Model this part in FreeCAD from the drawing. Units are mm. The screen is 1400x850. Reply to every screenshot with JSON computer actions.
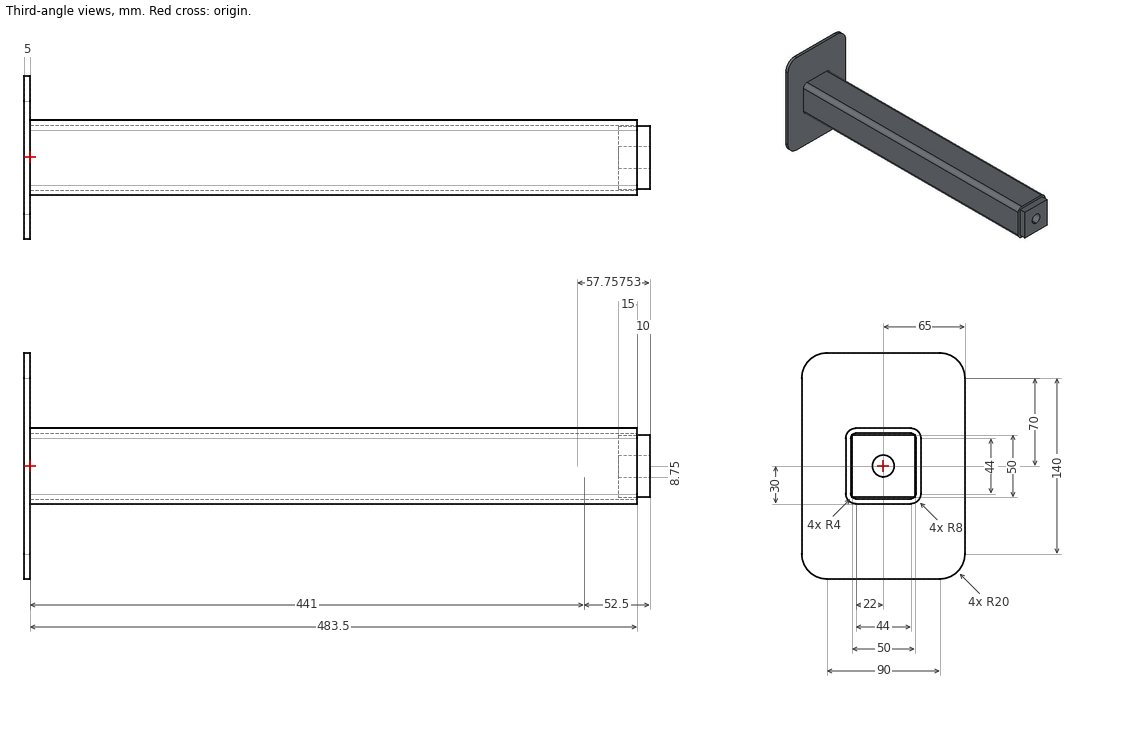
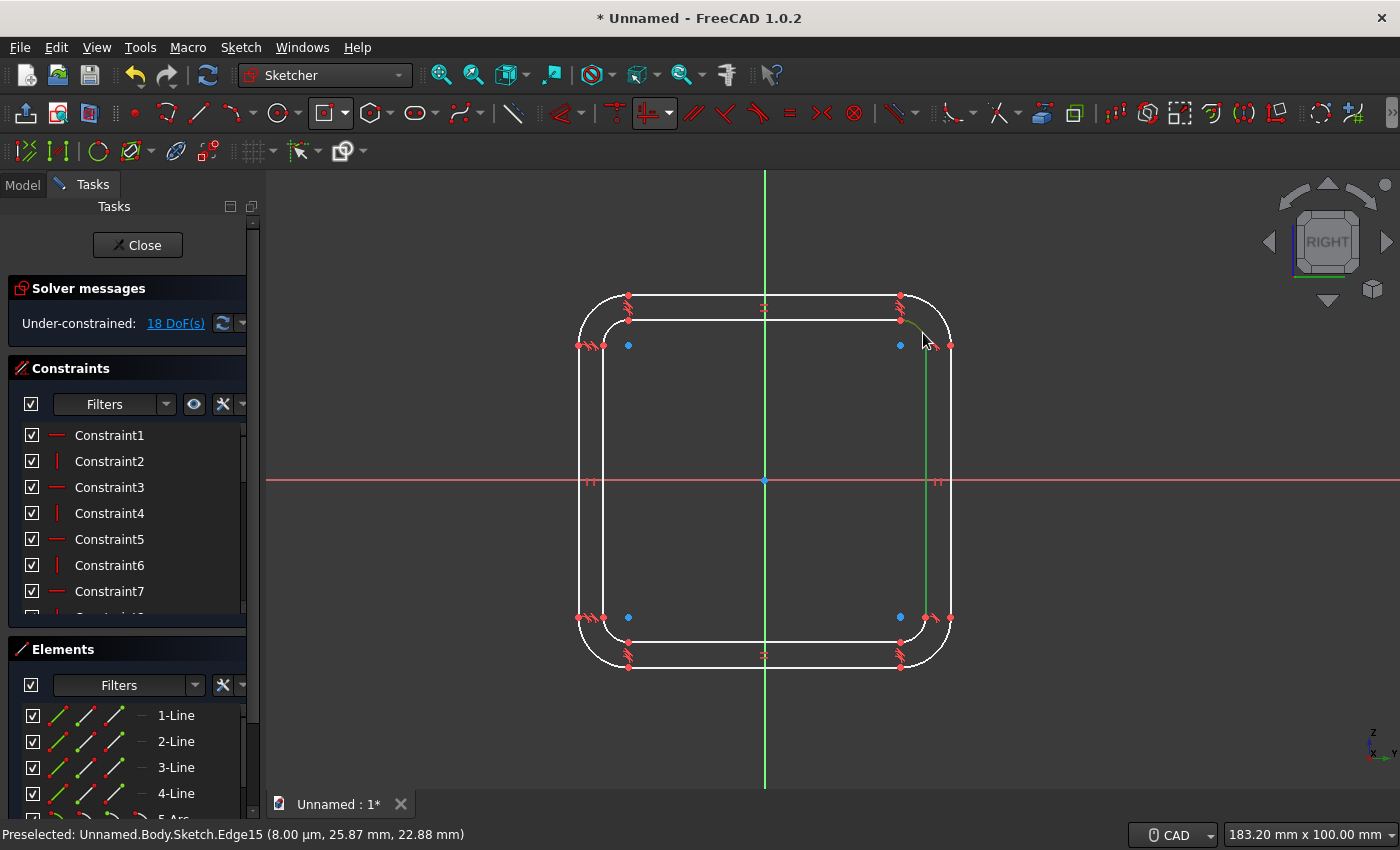
{"action": "key", "text": "t"}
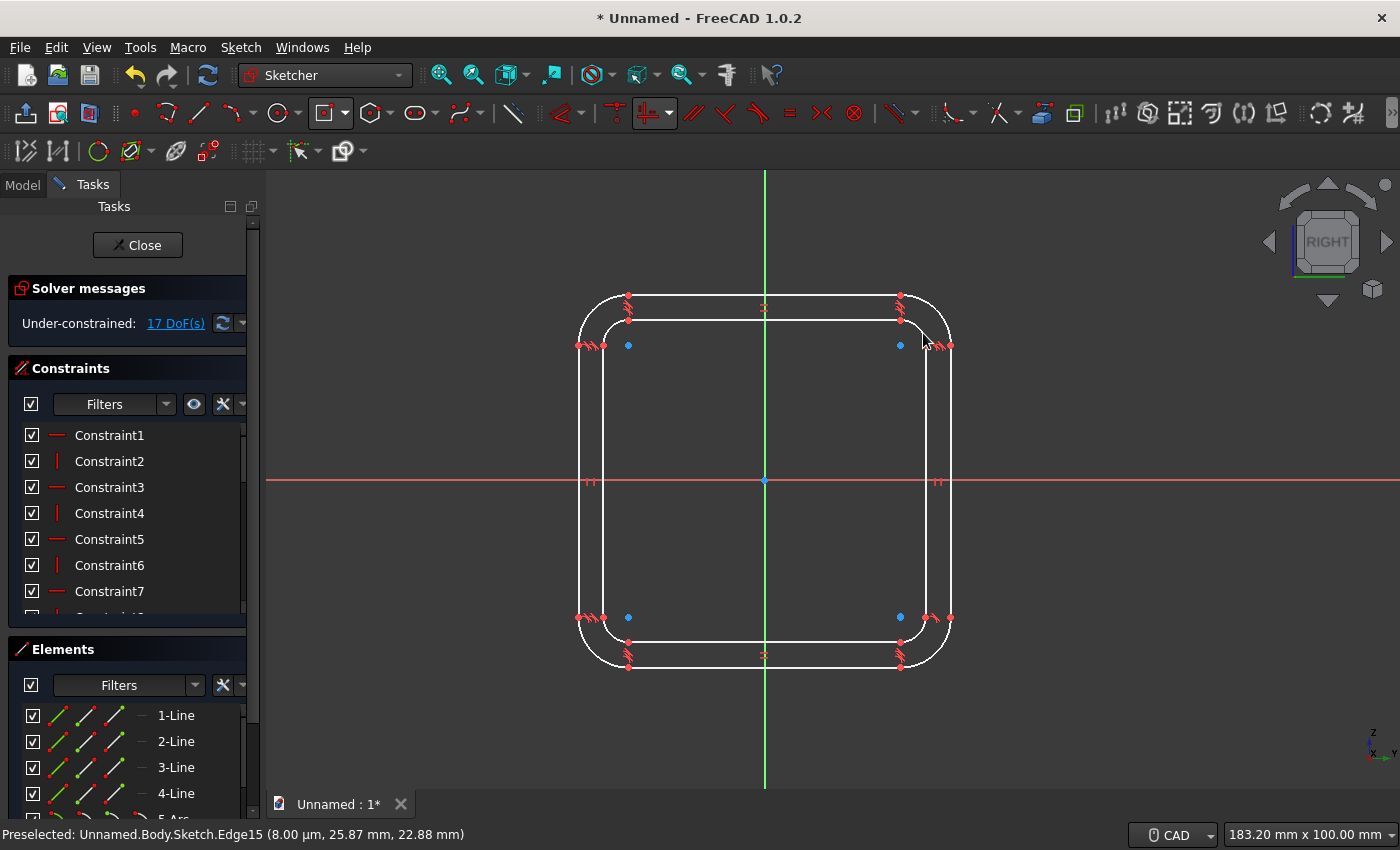
{"action": "left_click", "coordinate": [926, 427]}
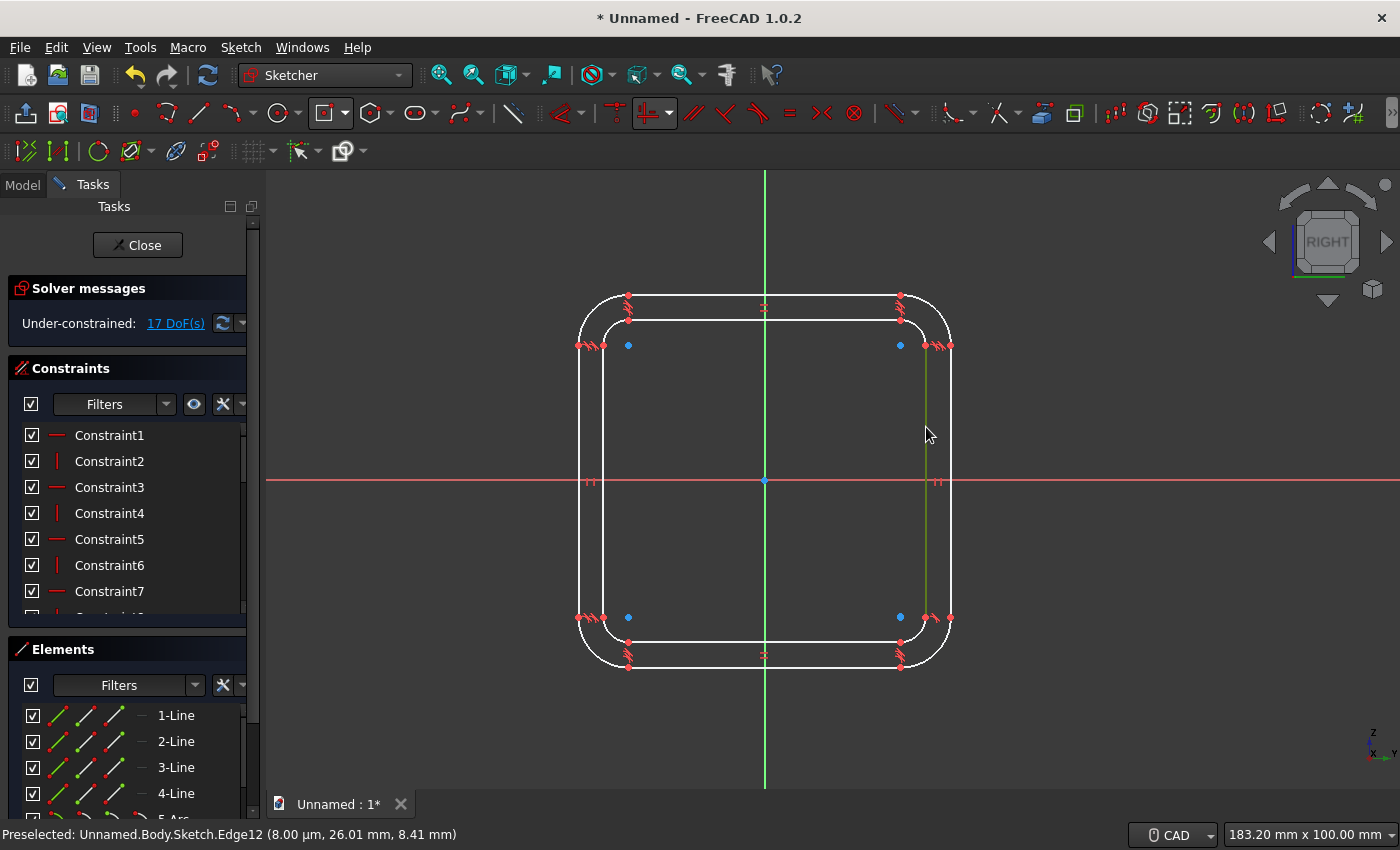
{"action": "left_click", "coordinate": [912, 639]}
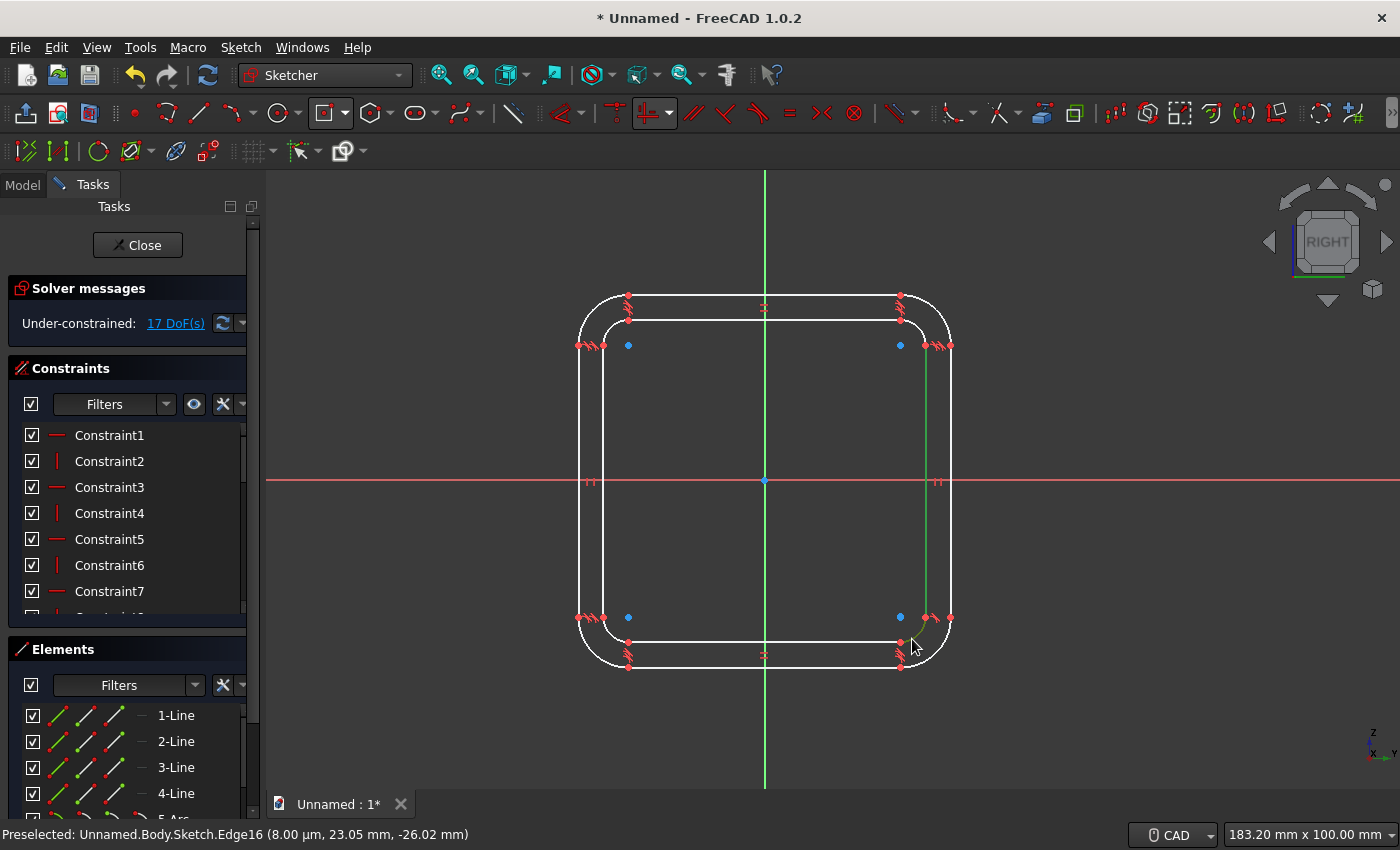
{"action": "left_click", "coordinate": [758, 114]}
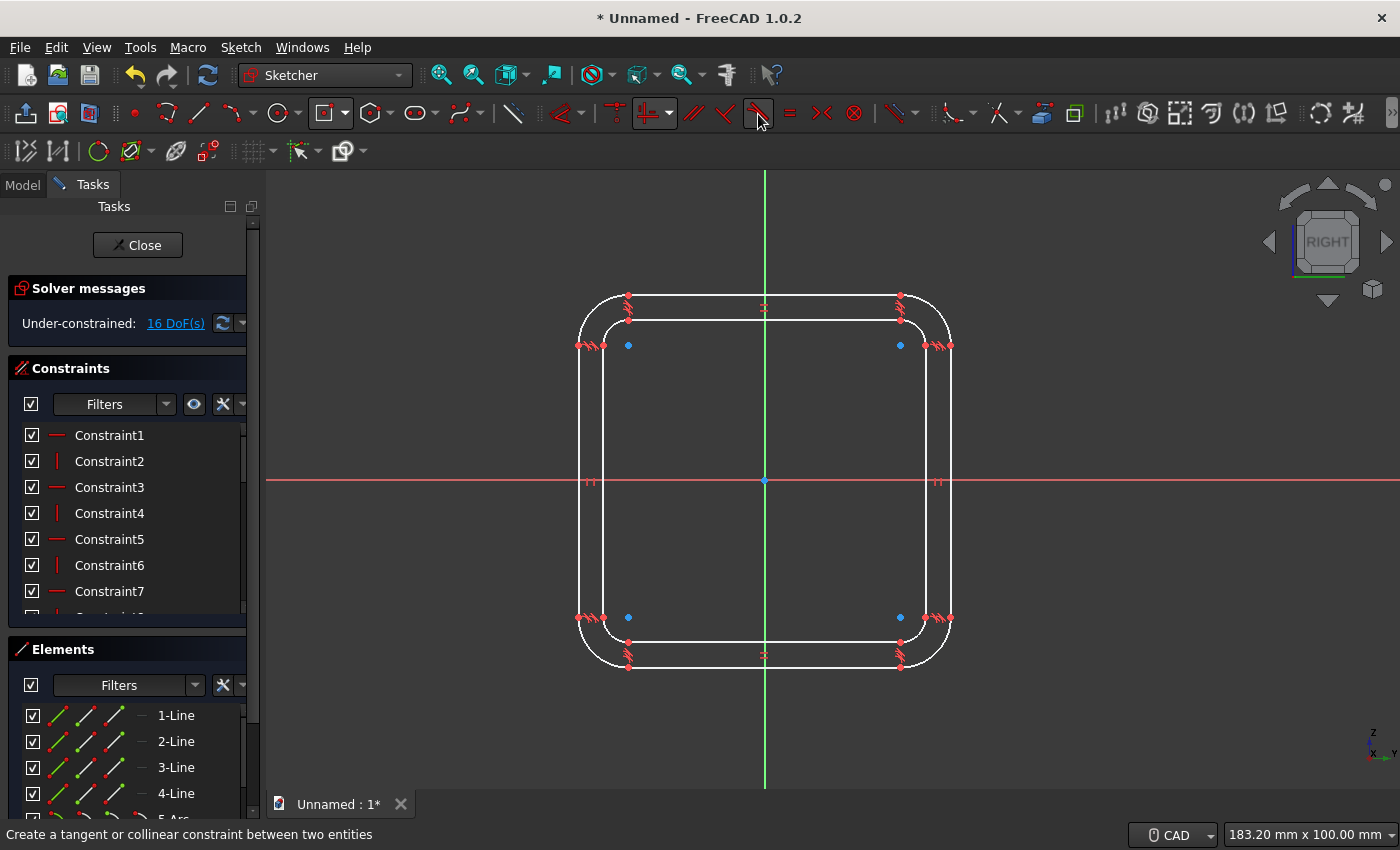
{"action": "left_click", "coordinate": [584, 640]}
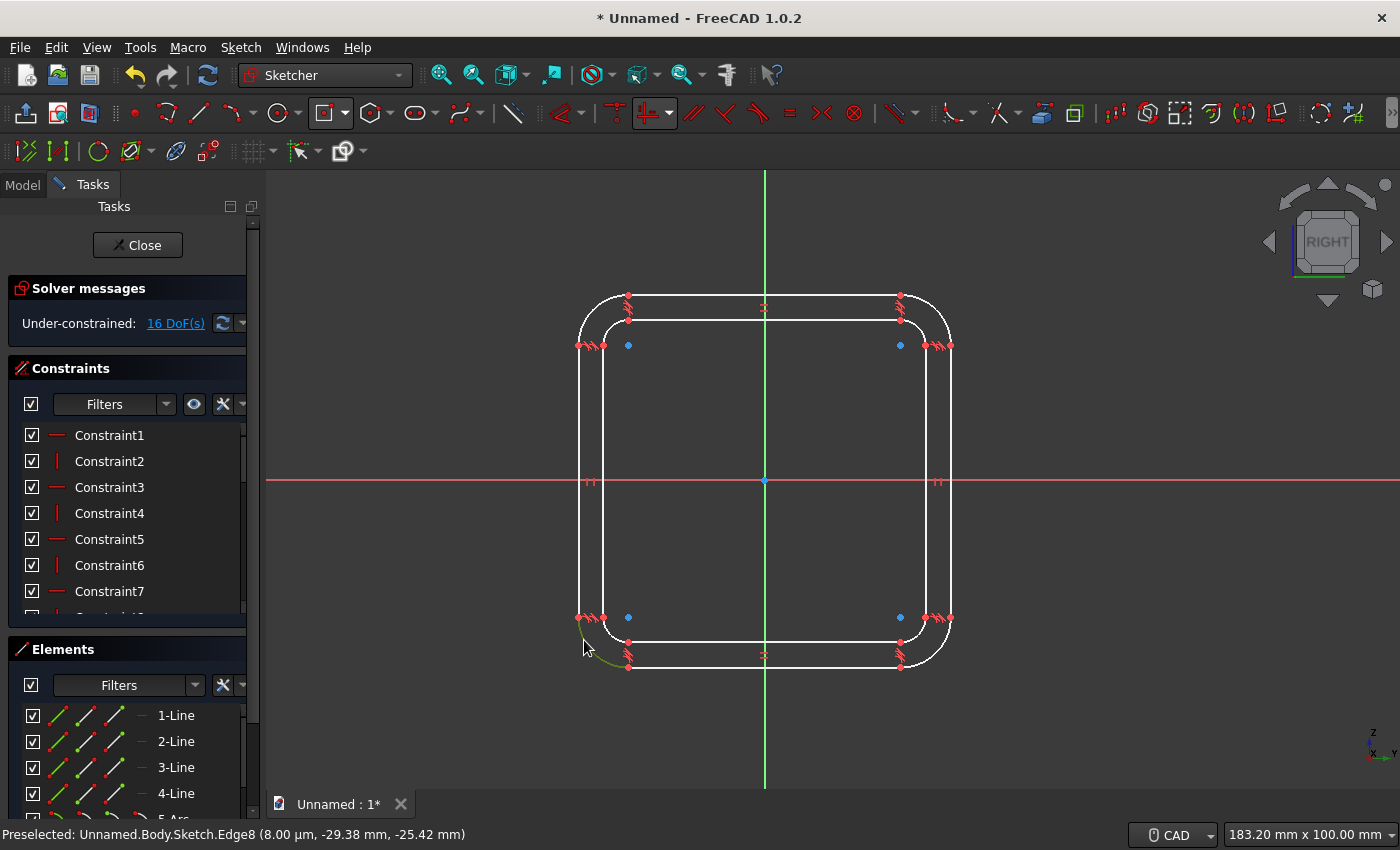
{"action": "left_click", "coordinate": [606, 629]}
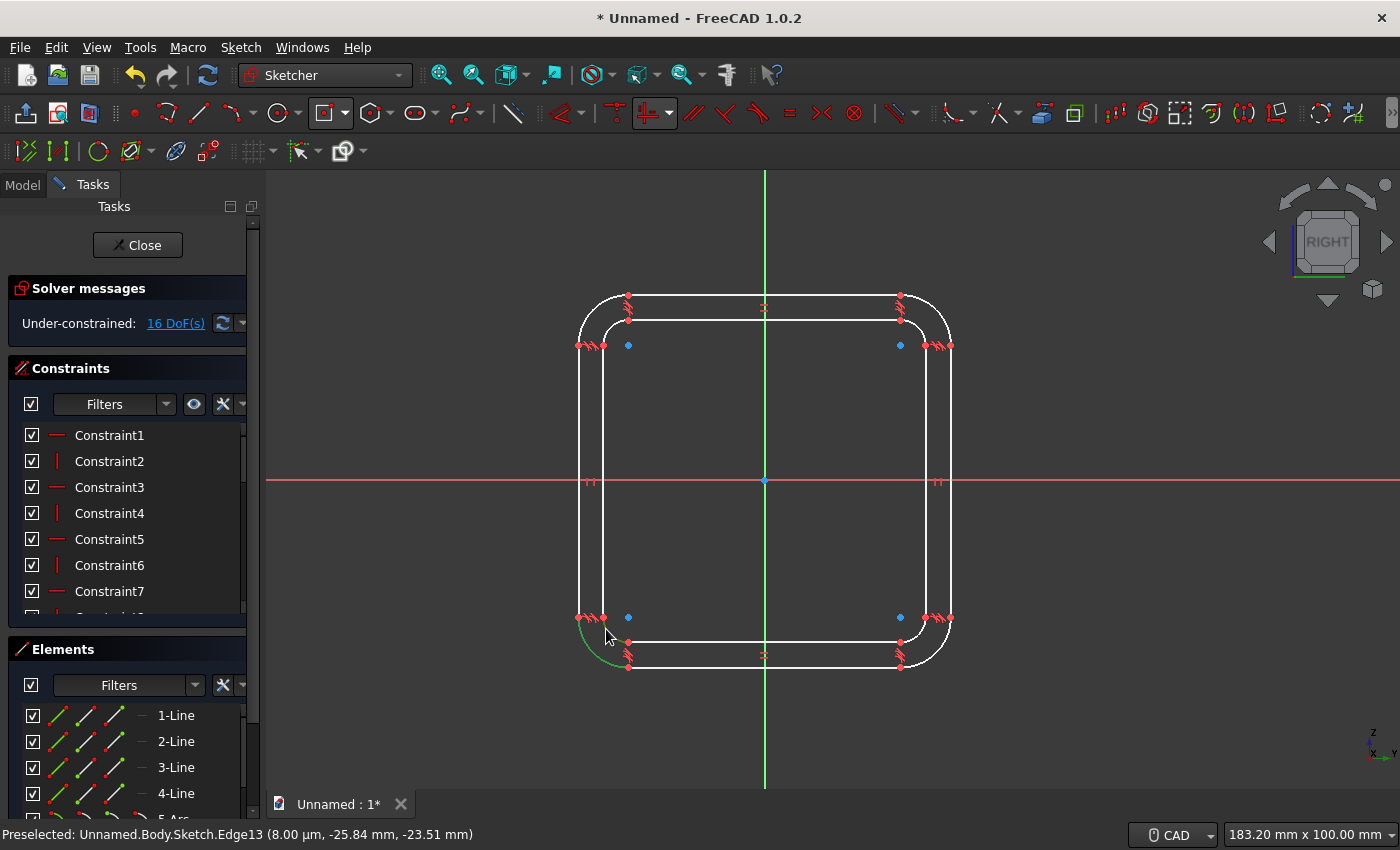
{"action": "left_click", "coordinate": [616, 114]}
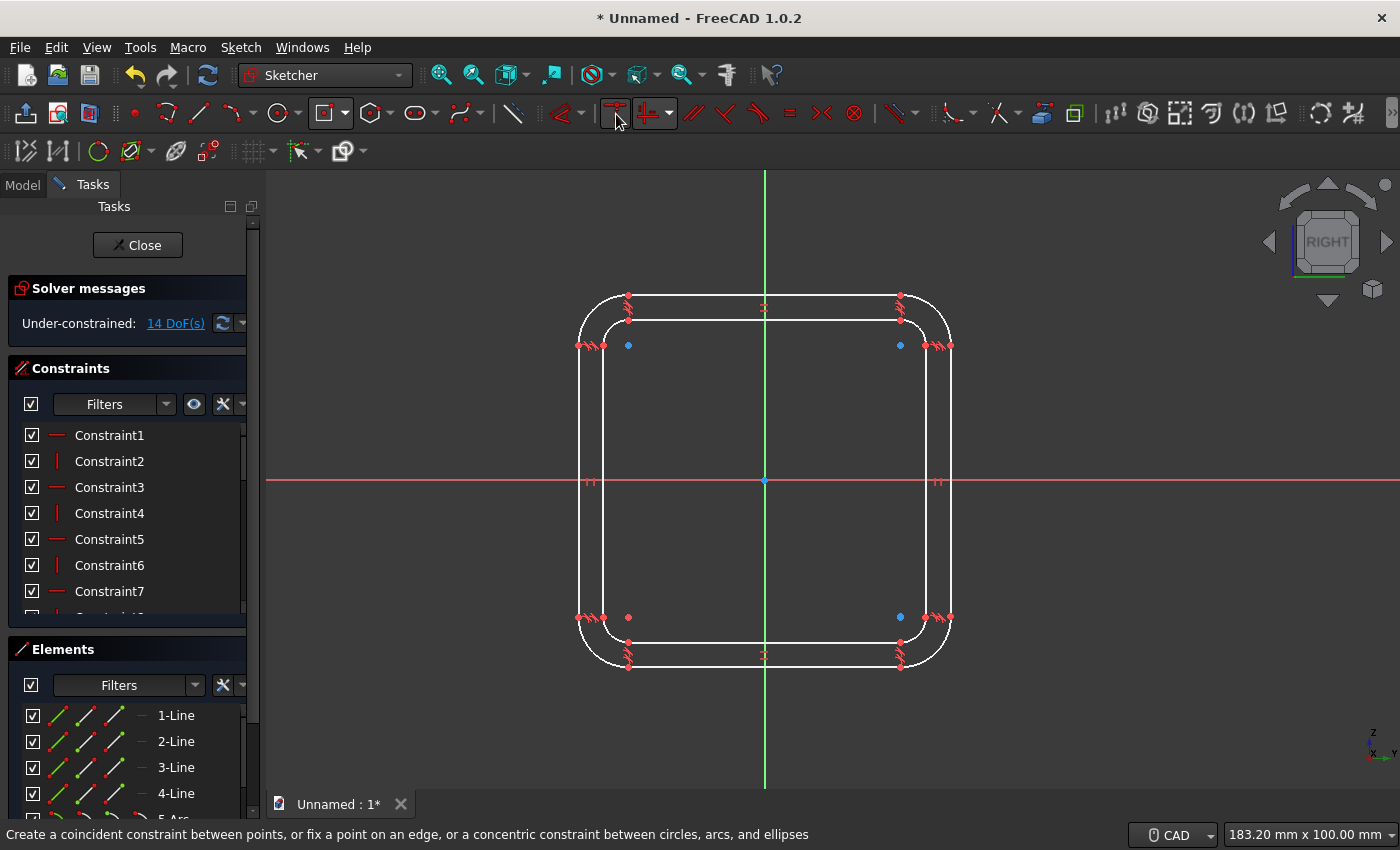
{"action": "left_click", "coordinate": [606, 300]}